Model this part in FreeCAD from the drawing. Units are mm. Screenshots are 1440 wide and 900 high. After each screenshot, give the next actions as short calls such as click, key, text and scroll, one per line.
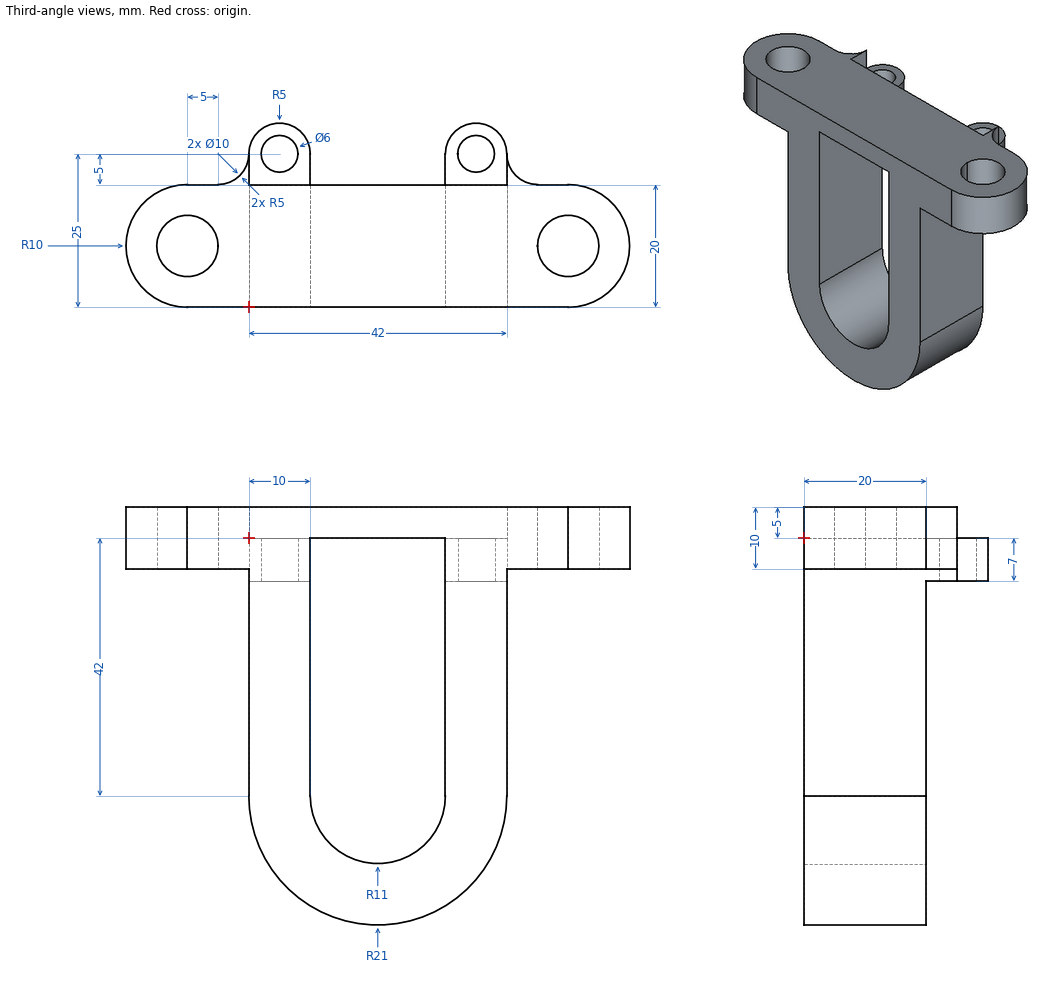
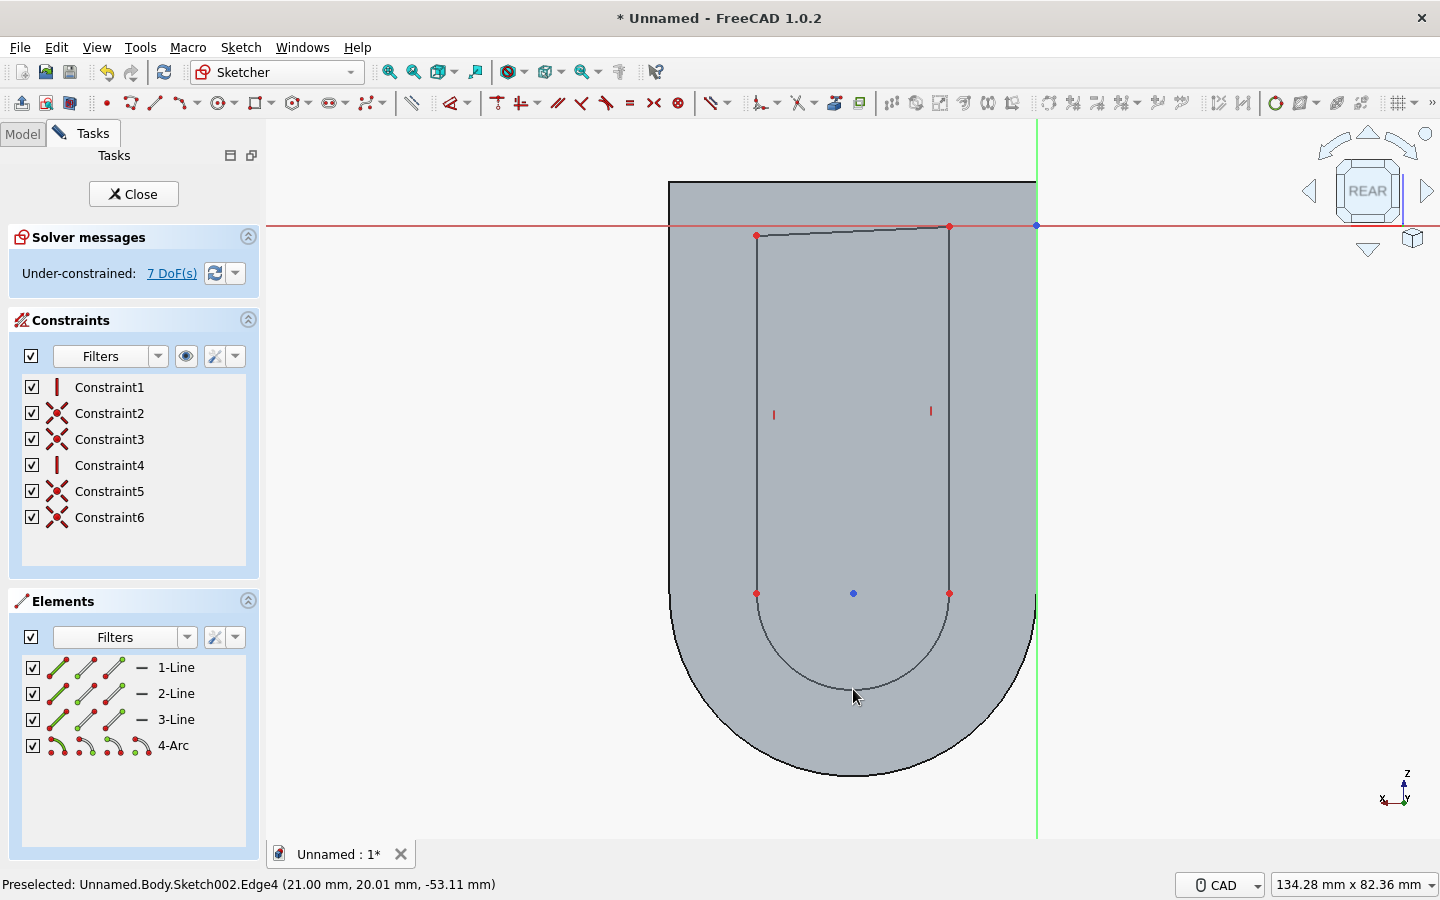
click(949, 484)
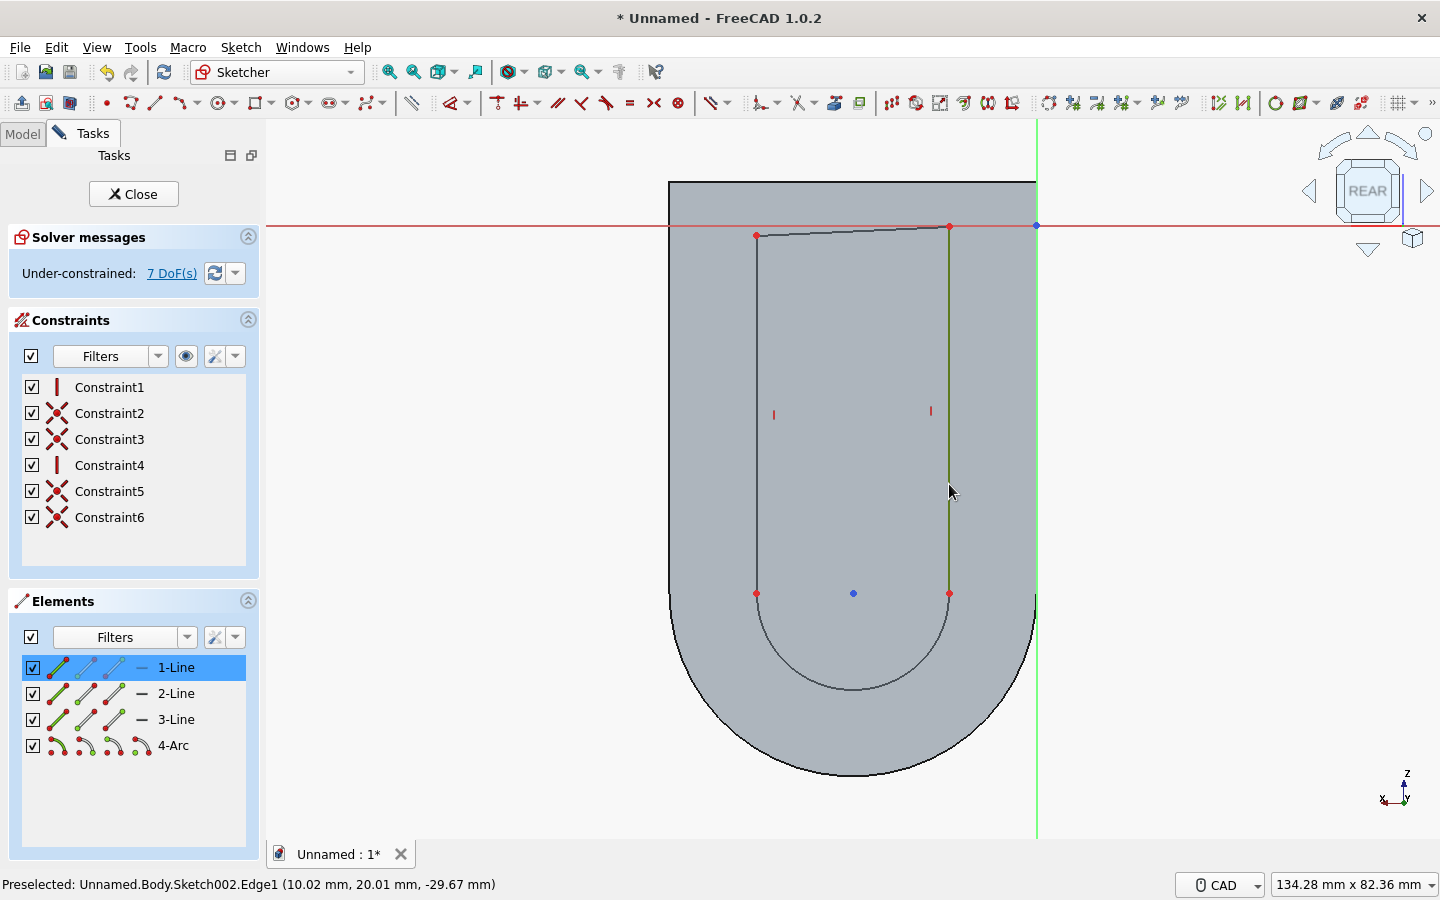
click(797, 672)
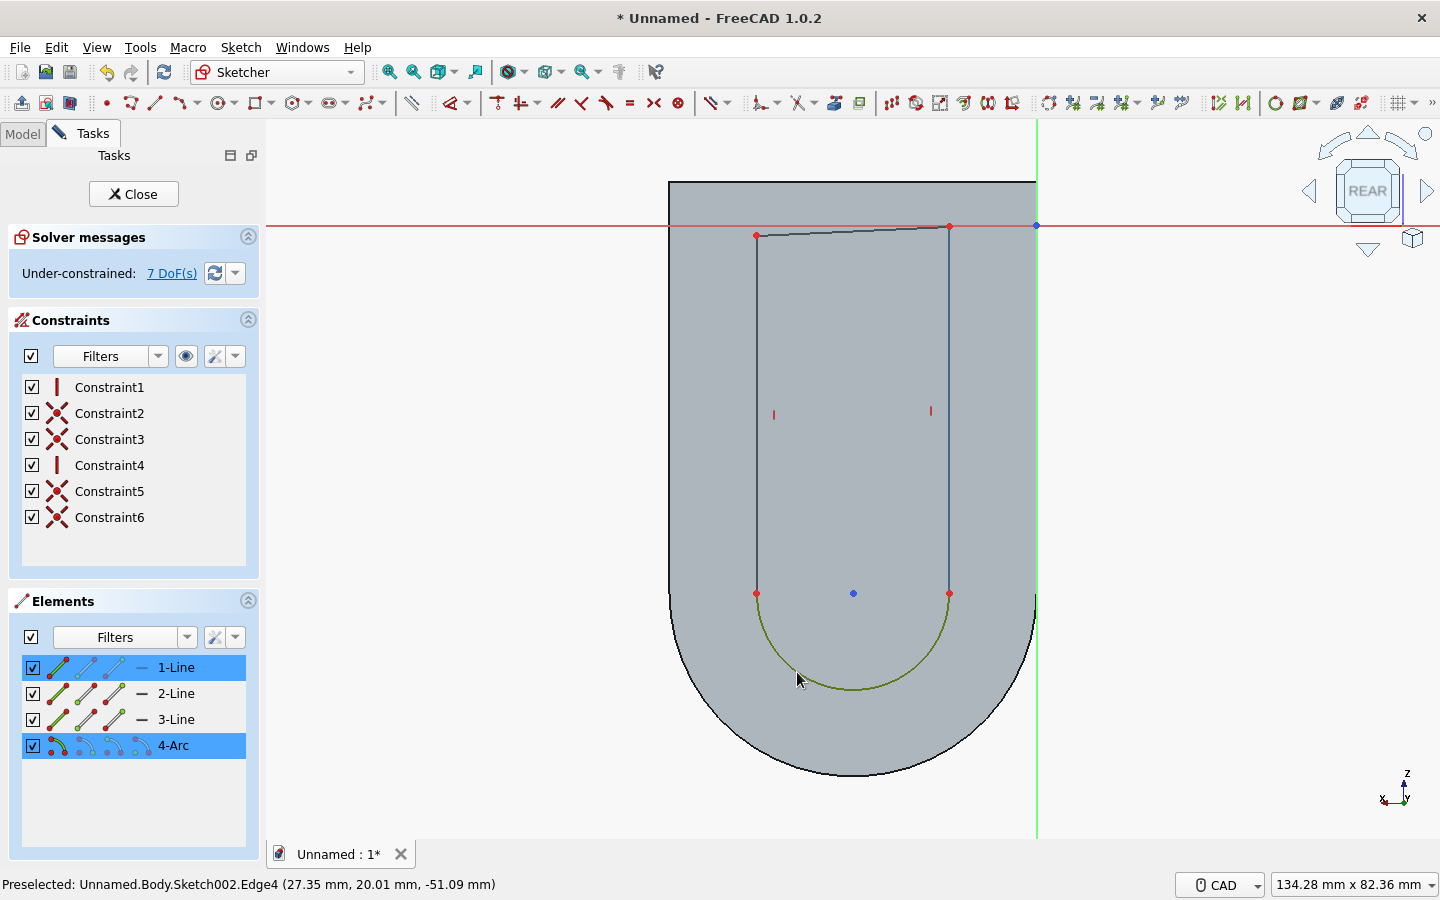
click(606, 104)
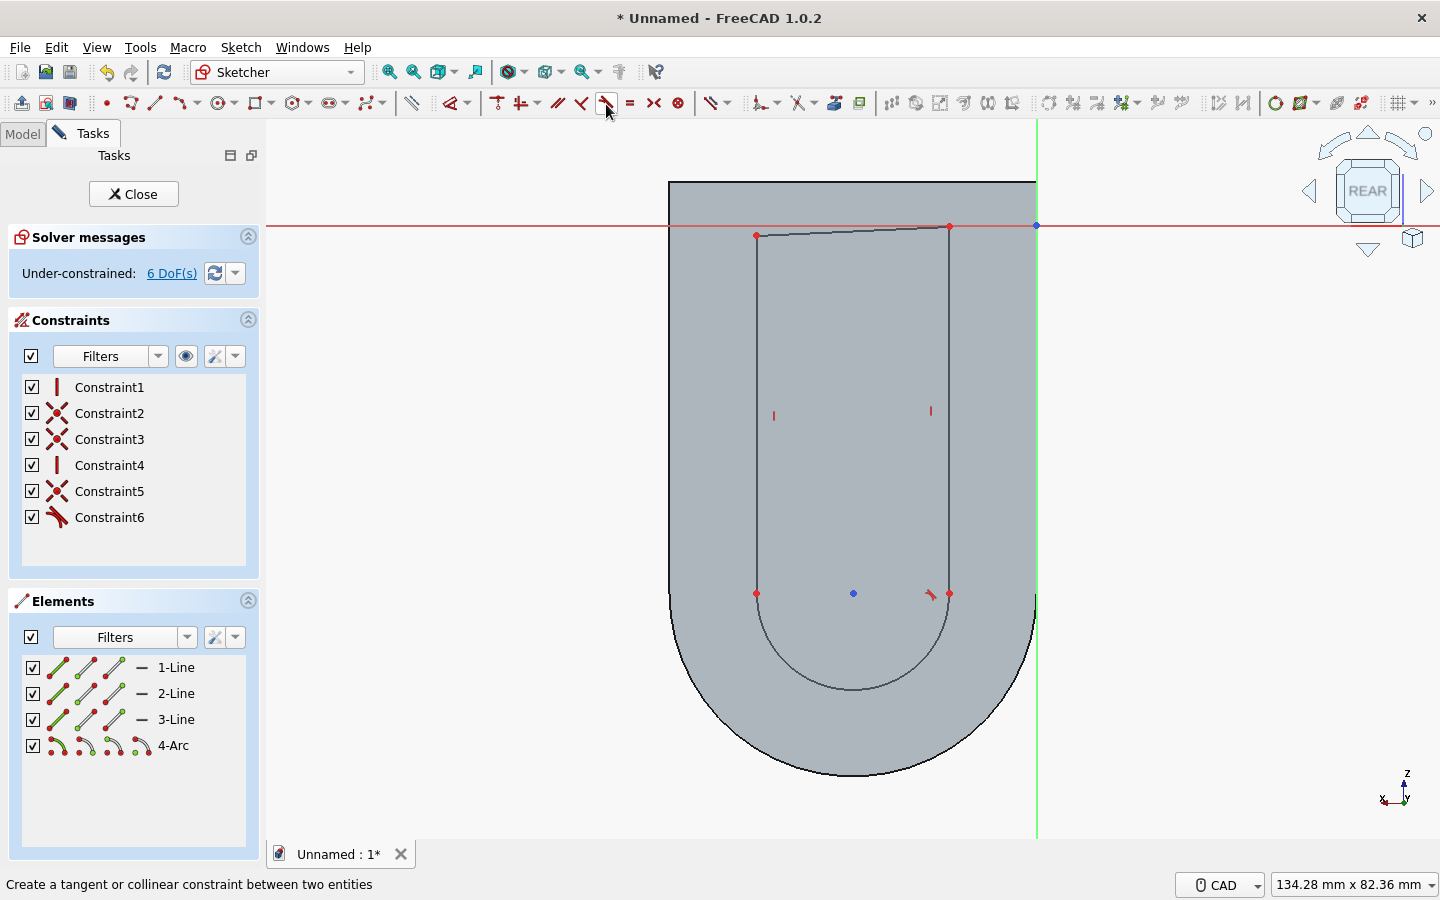
click(757, 343)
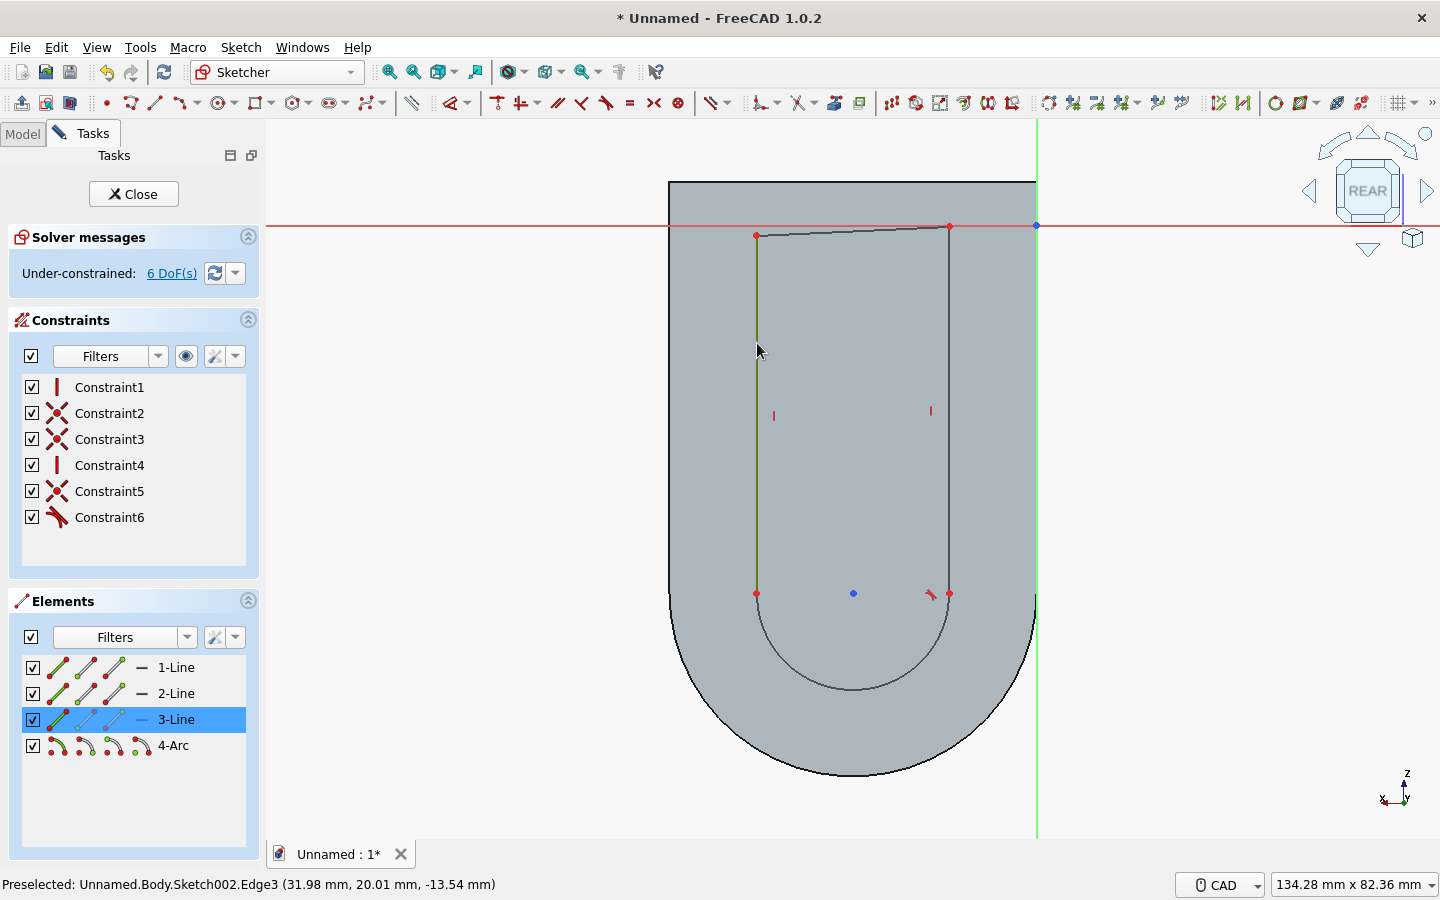
click(797, 672)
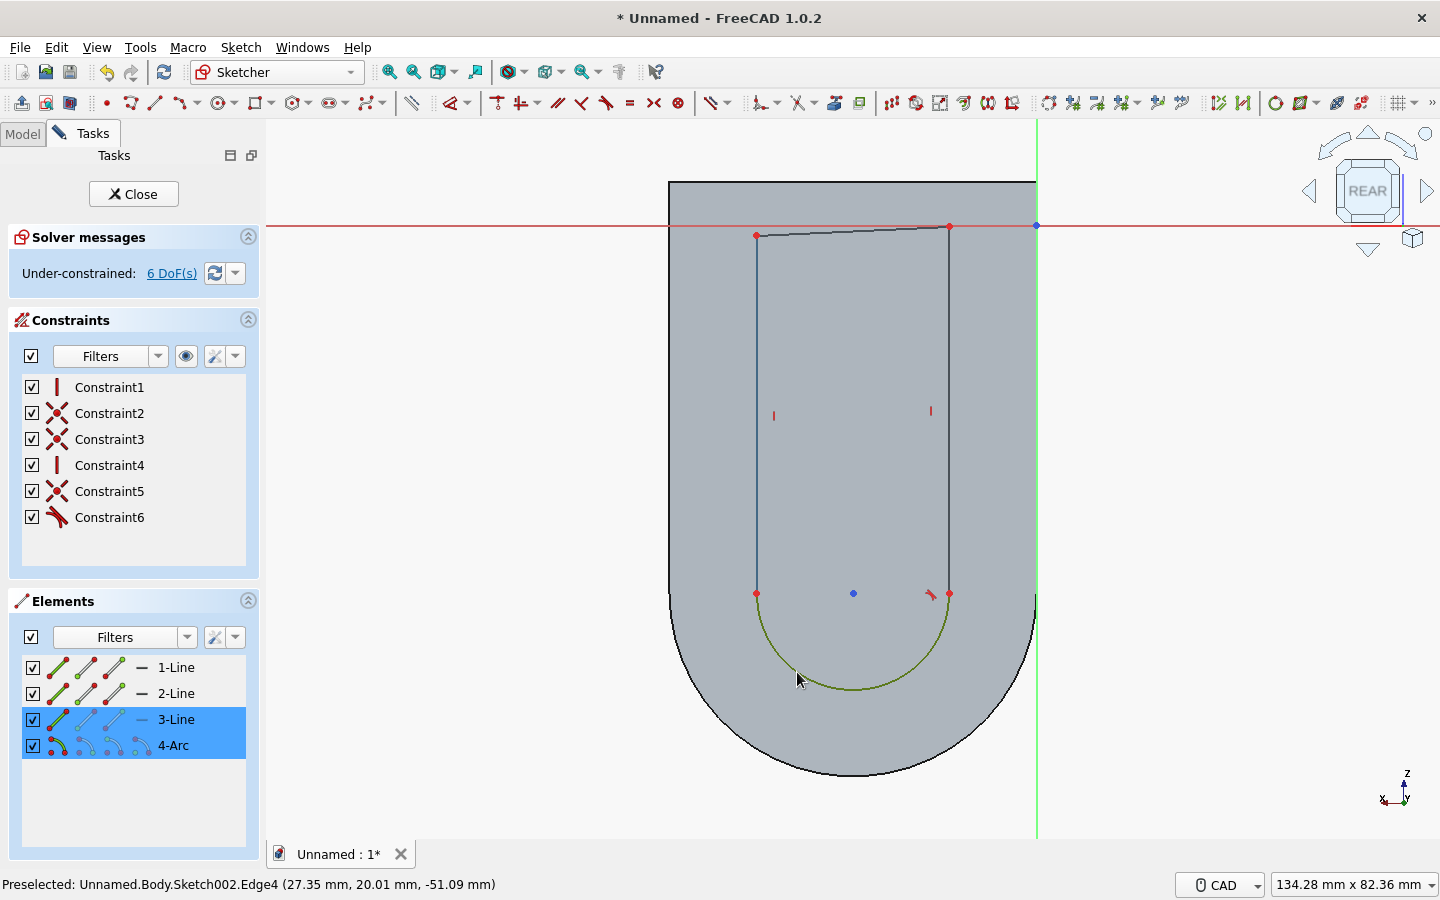
click(606, 104)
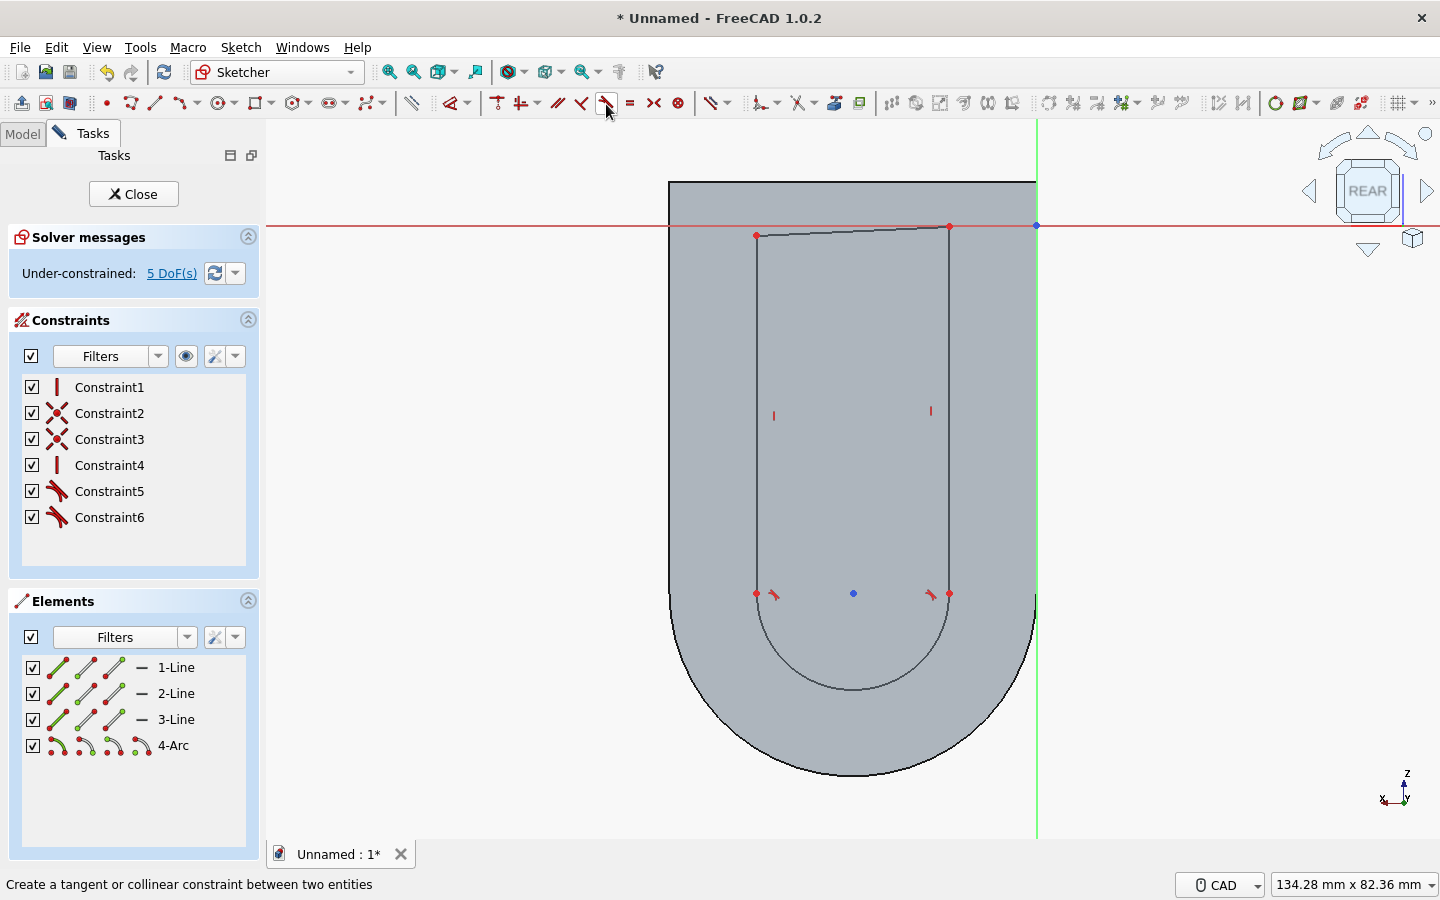
click(911, 229)